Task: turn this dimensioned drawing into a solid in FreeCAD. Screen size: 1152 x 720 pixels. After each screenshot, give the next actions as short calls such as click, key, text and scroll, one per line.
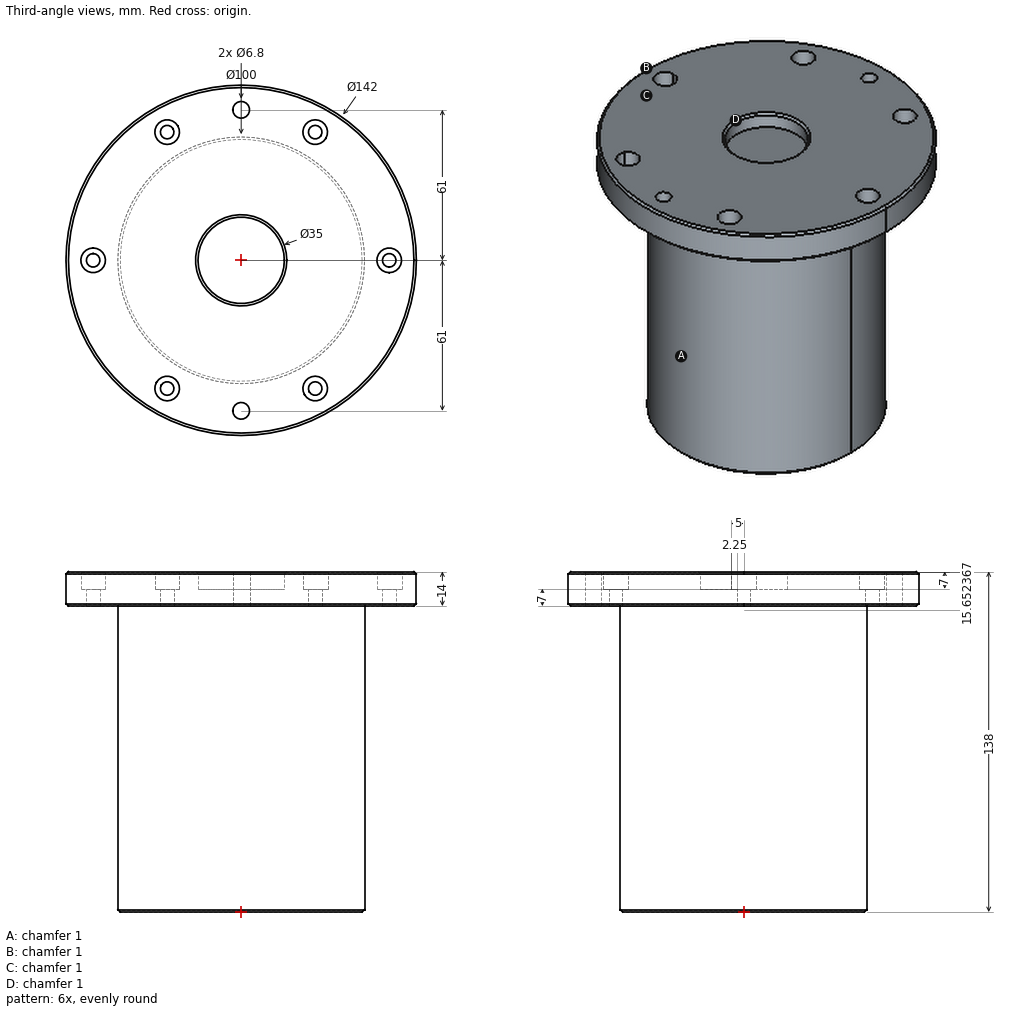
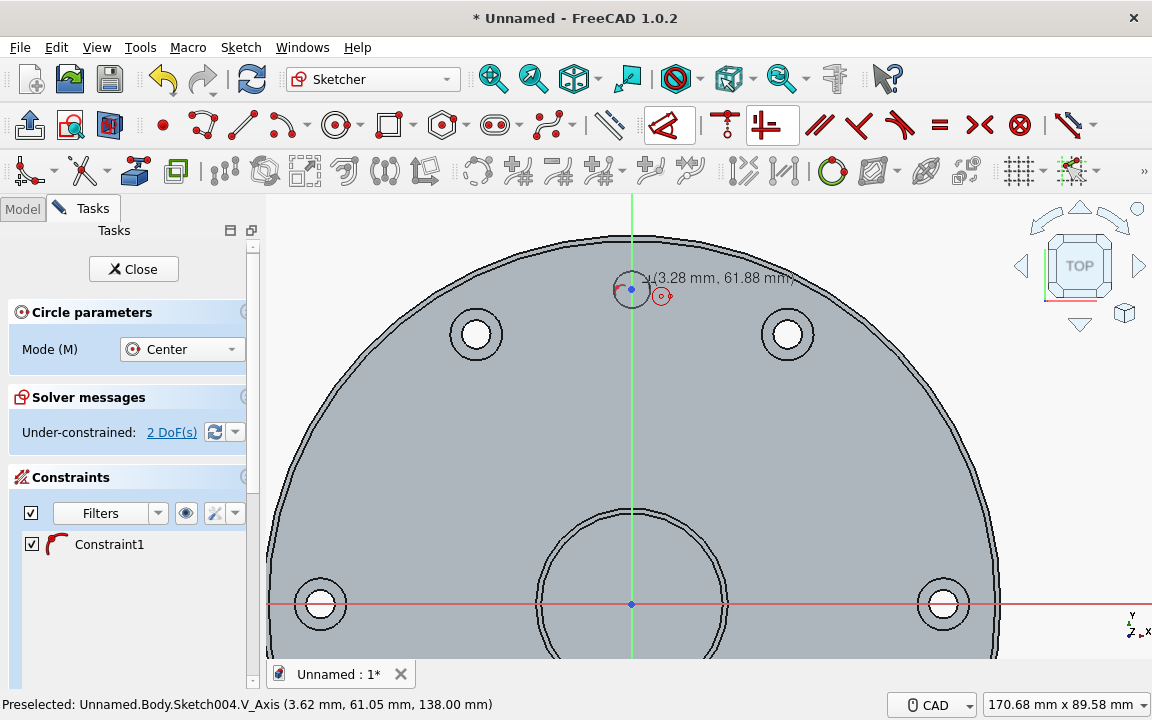
scroll(647, 282, down, 4)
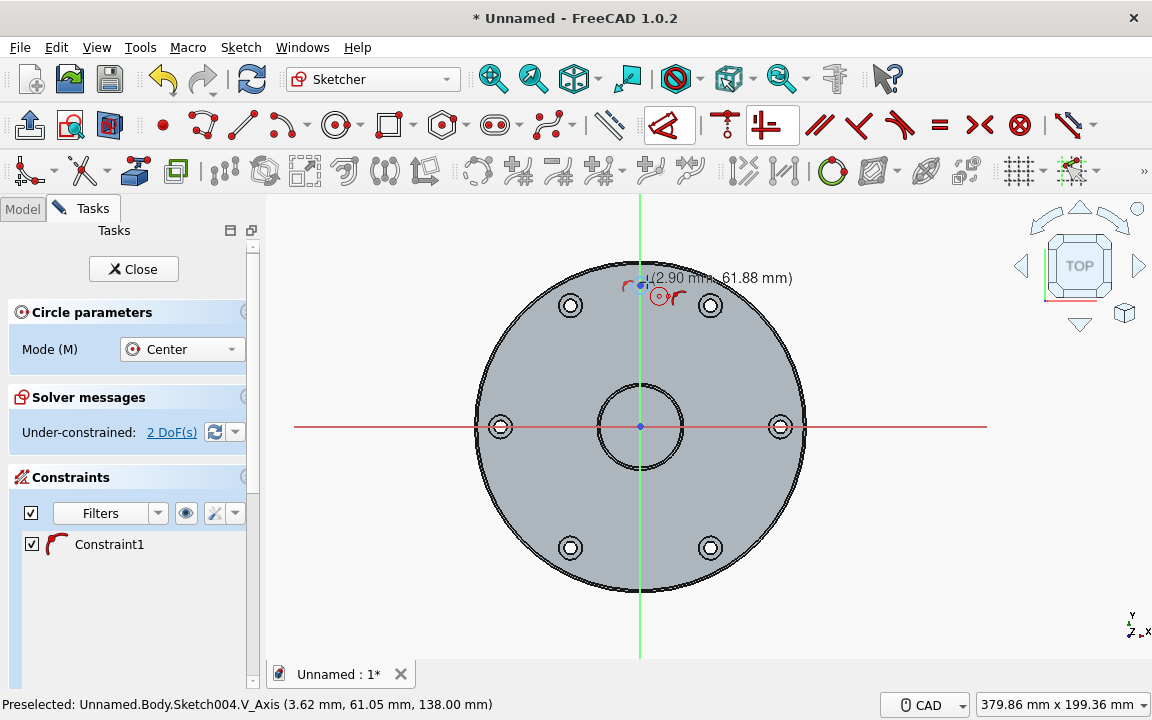
scroll(640, 569, up, 6)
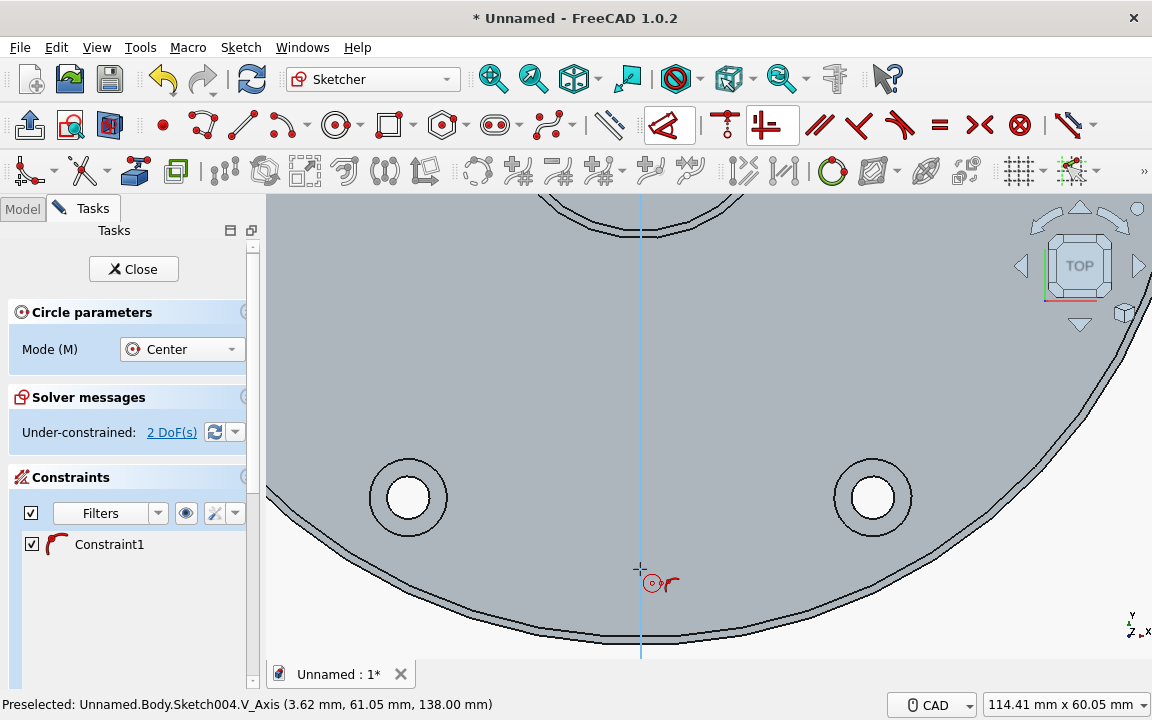
scroll(640, 569, down, 6)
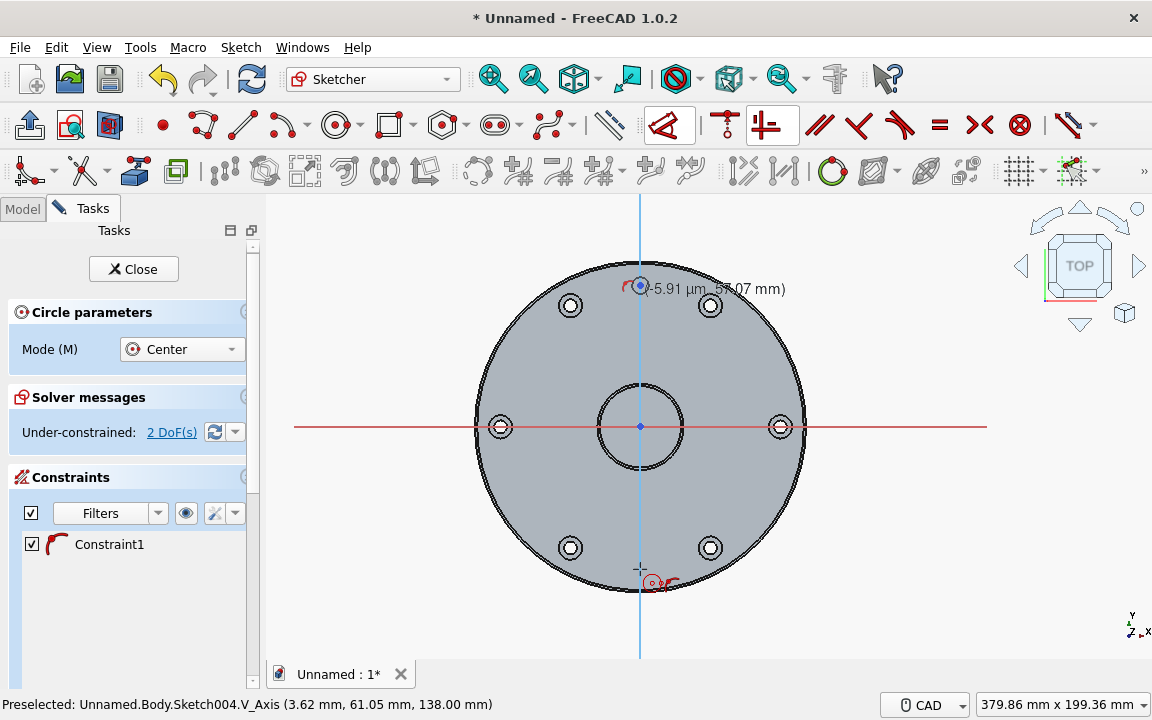
click(640, 569)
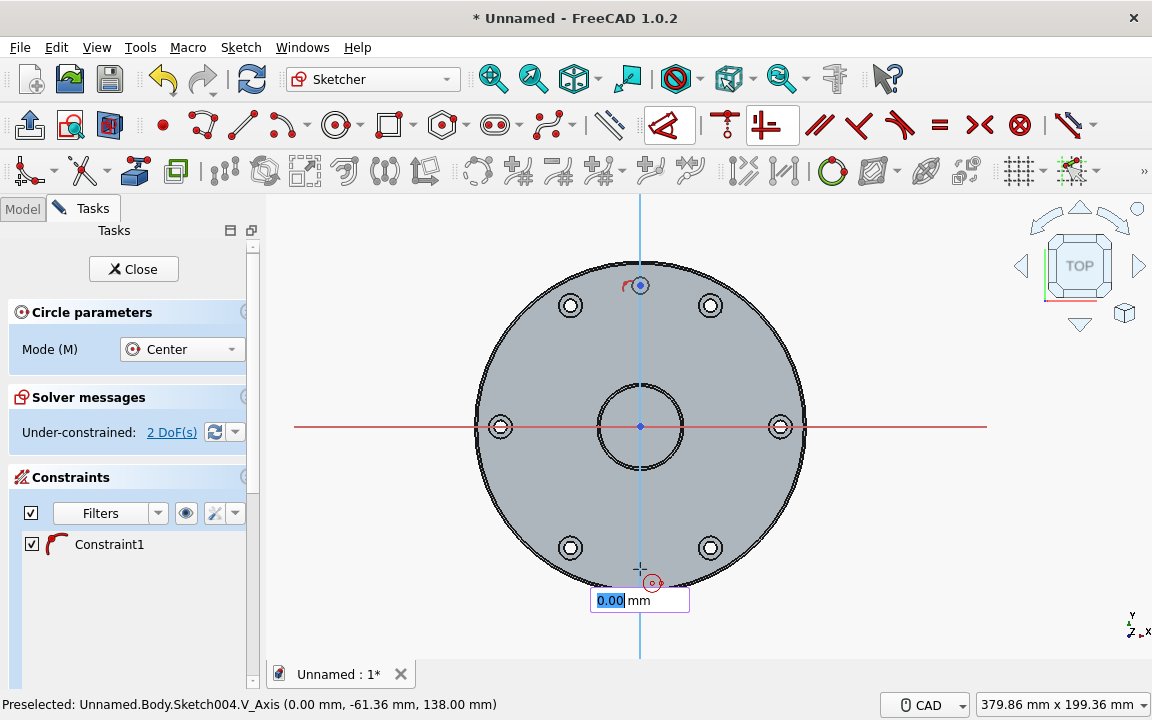
scroll(648, 566, up, 4)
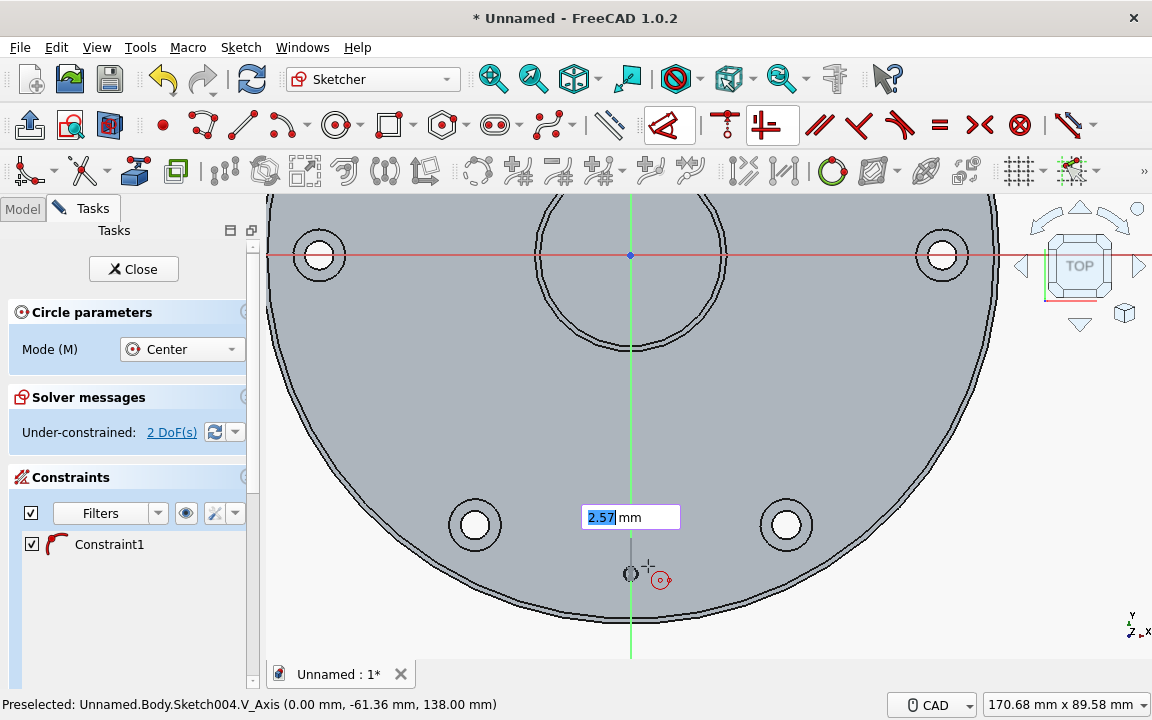
click(647, 566)
key(Escape)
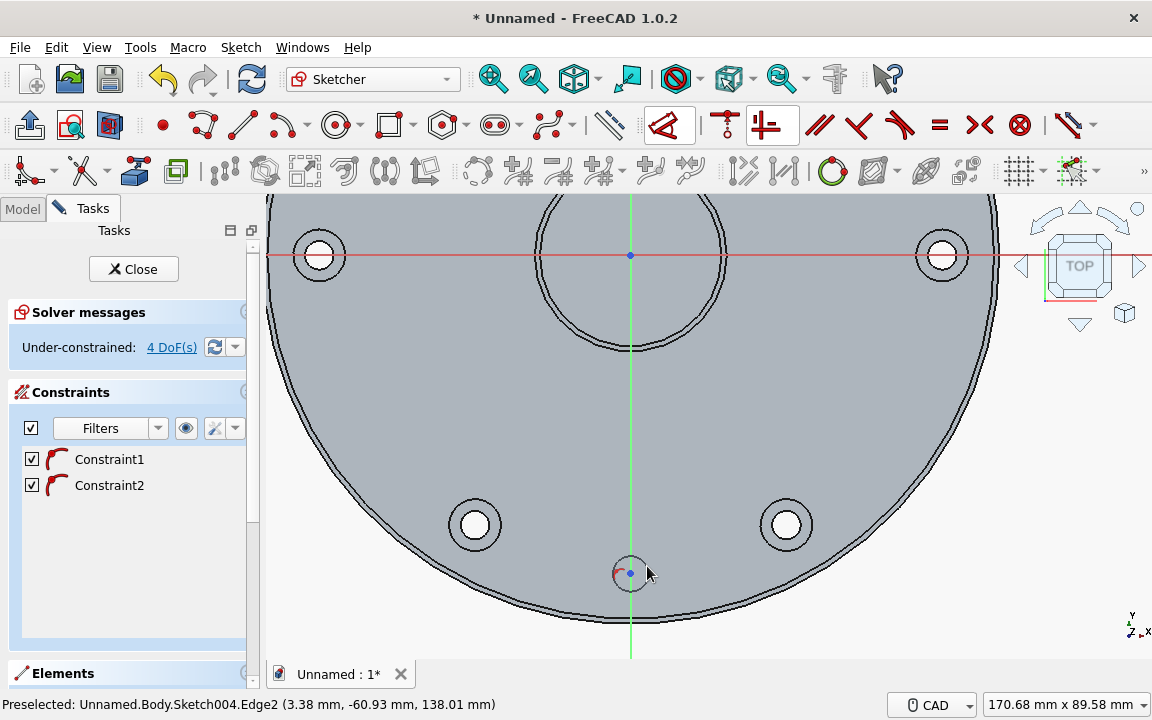
scroll(648, 566, down, 4)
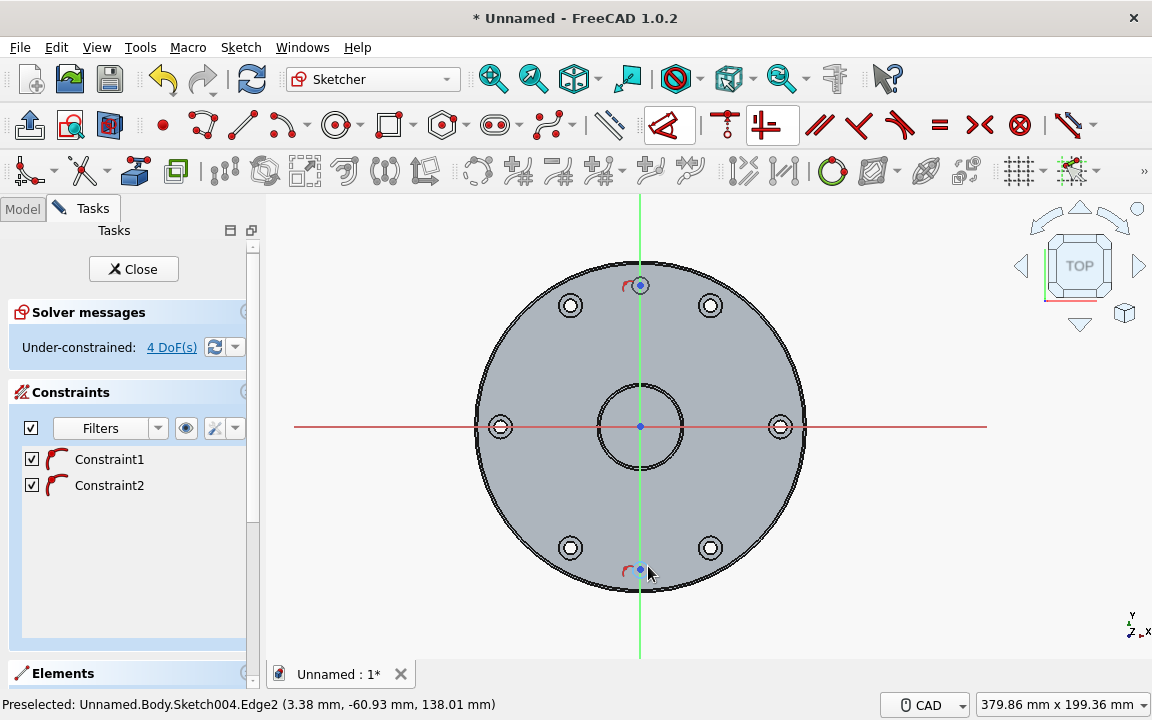
scroll(646, 280, up, 5)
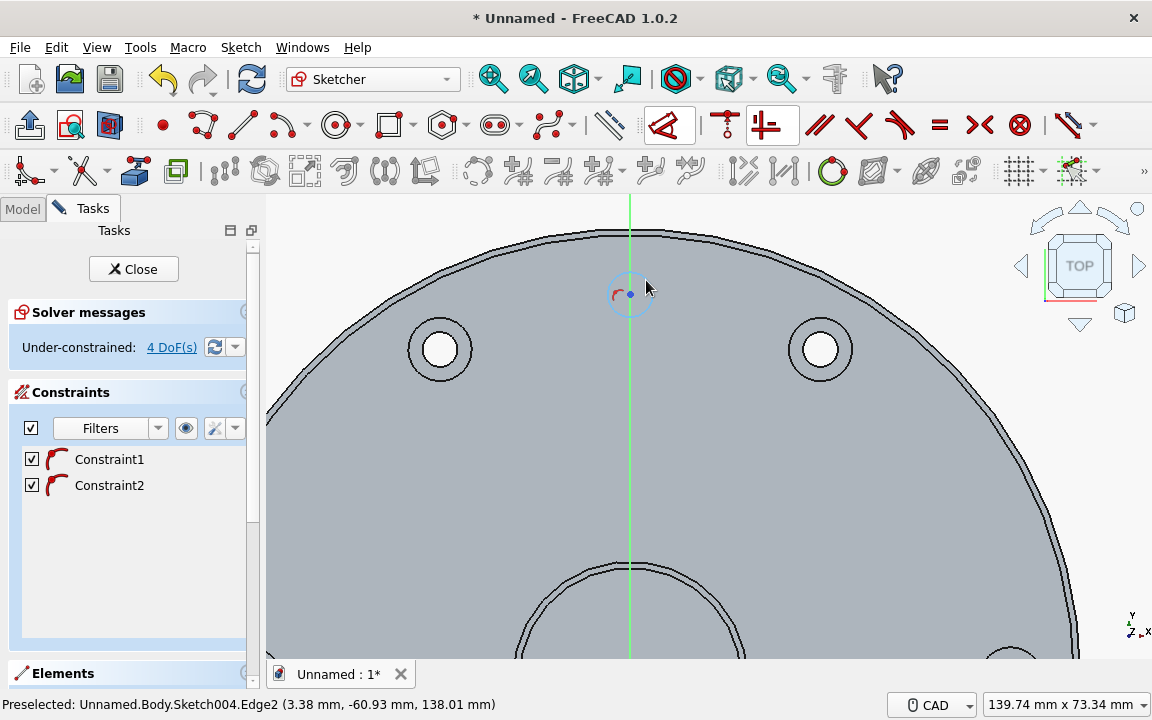
click(646, 279)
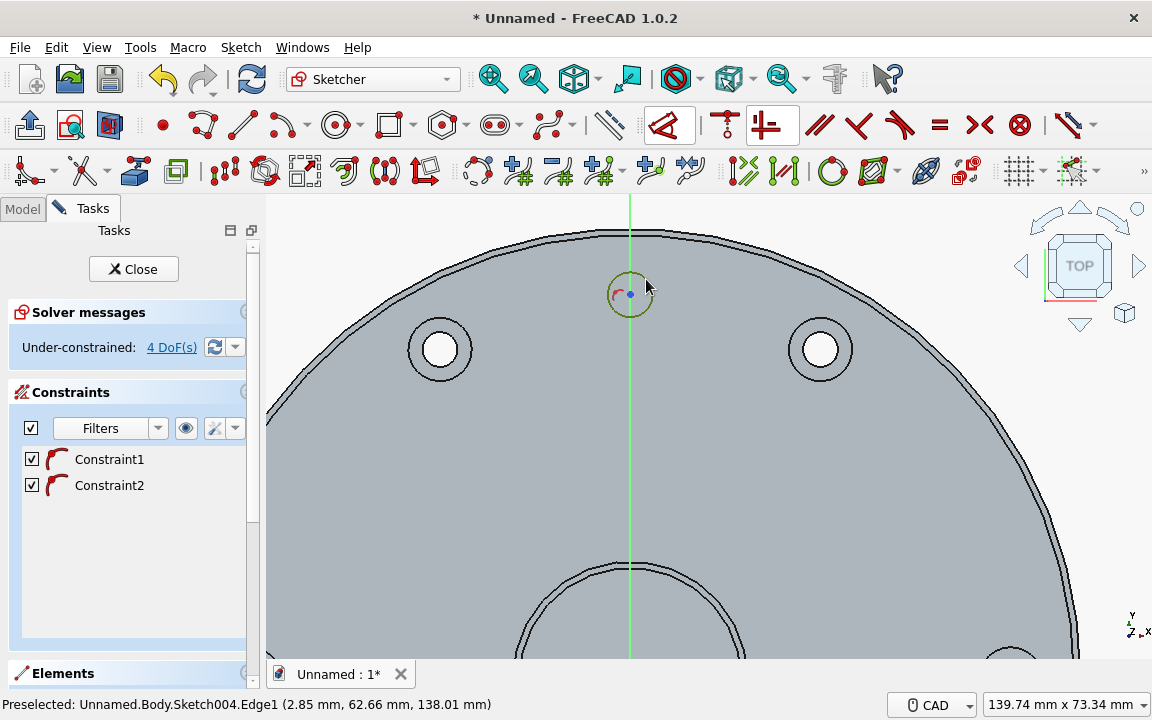
scroll(646, 280, down, 5)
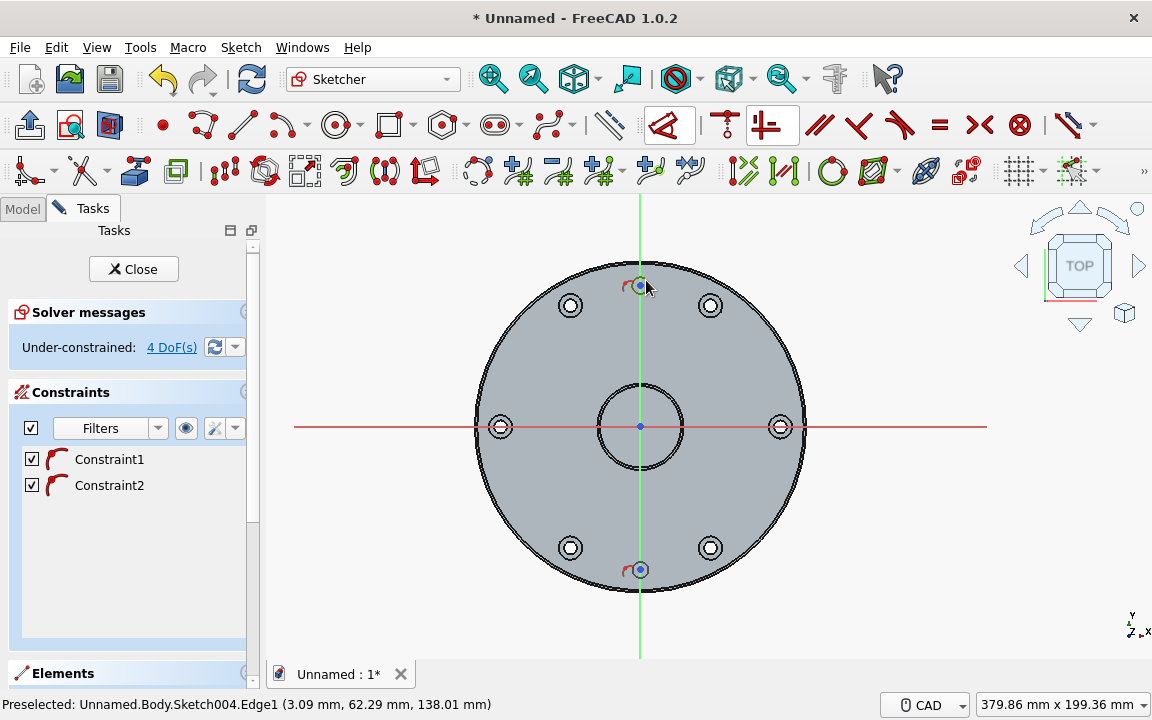
scroll(646, 564, up, 5)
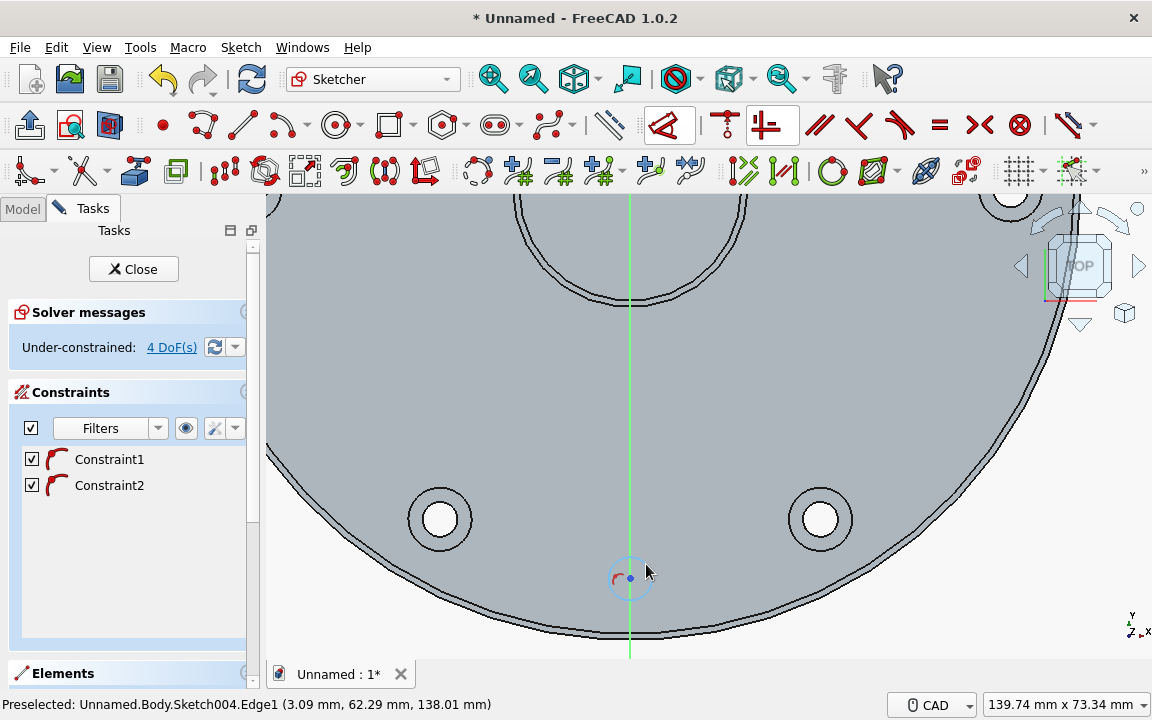
click(645, 564)